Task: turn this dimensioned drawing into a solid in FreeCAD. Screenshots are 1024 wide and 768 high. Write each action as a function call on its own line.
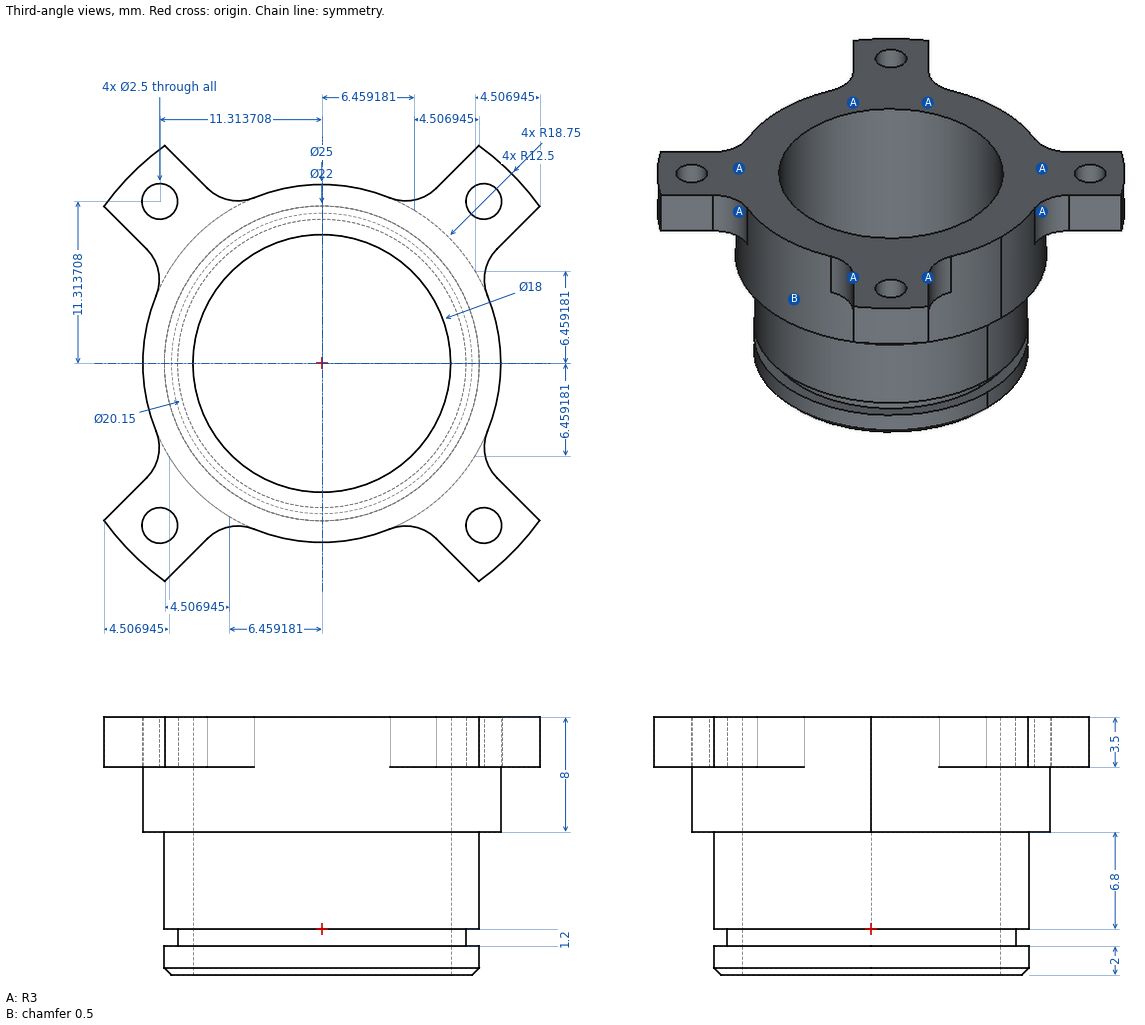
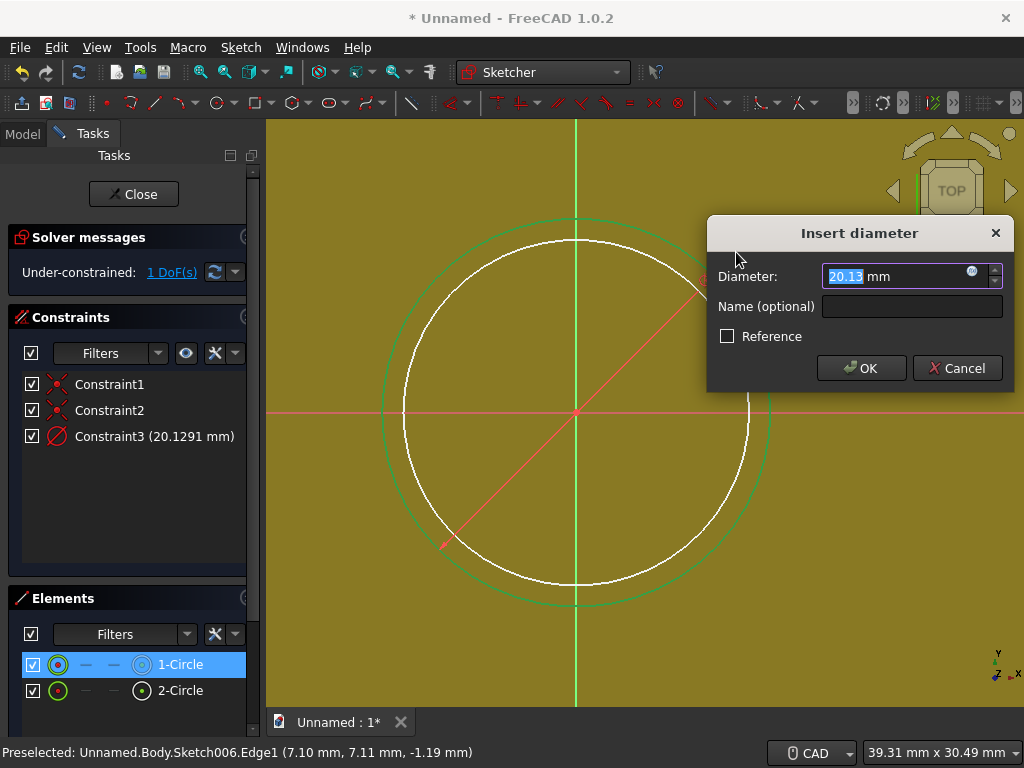
text(20.15)
key(Return)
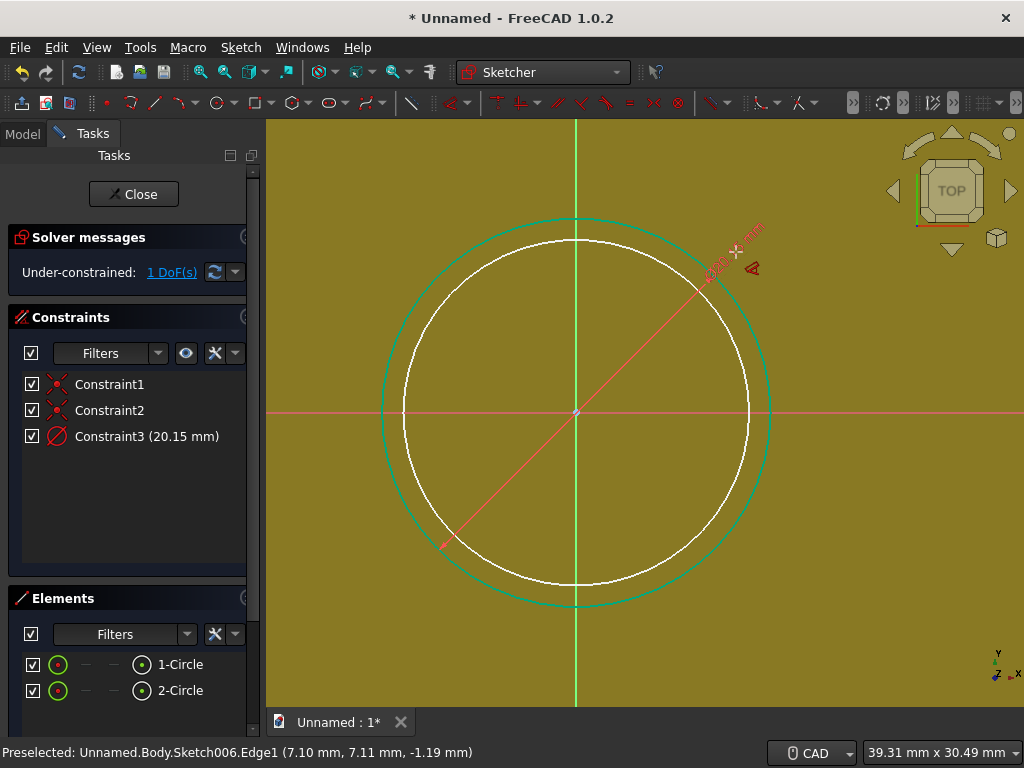
click(698, 290)
click(795, 348)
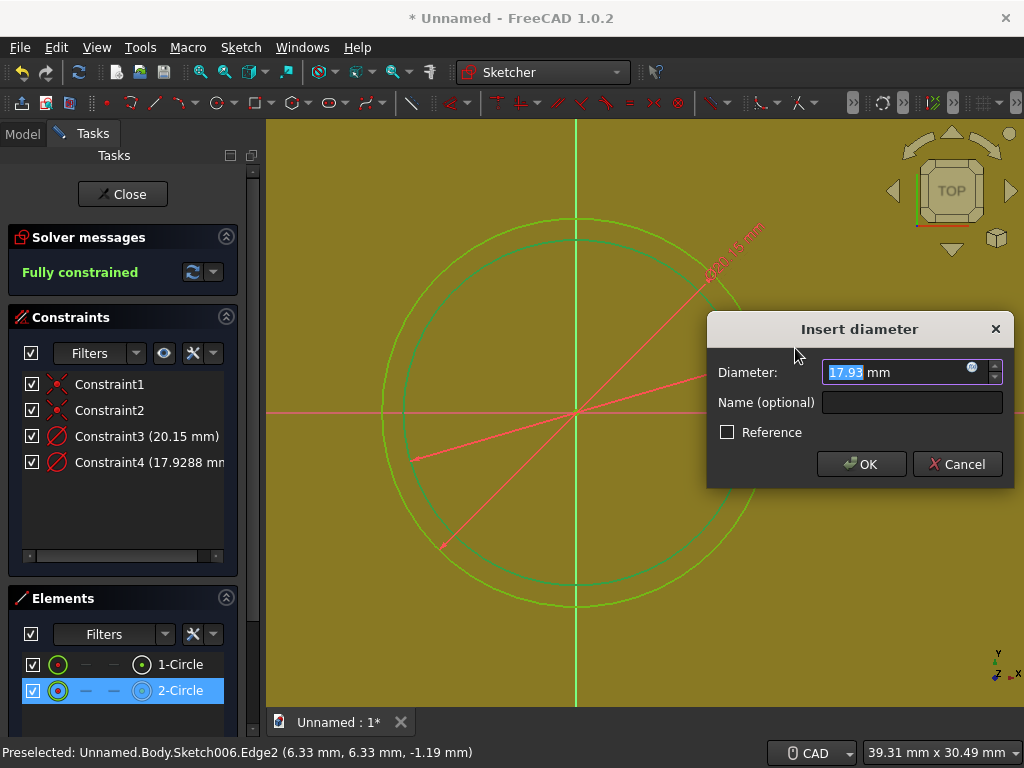
text(18)
key(Return)
key(Escape)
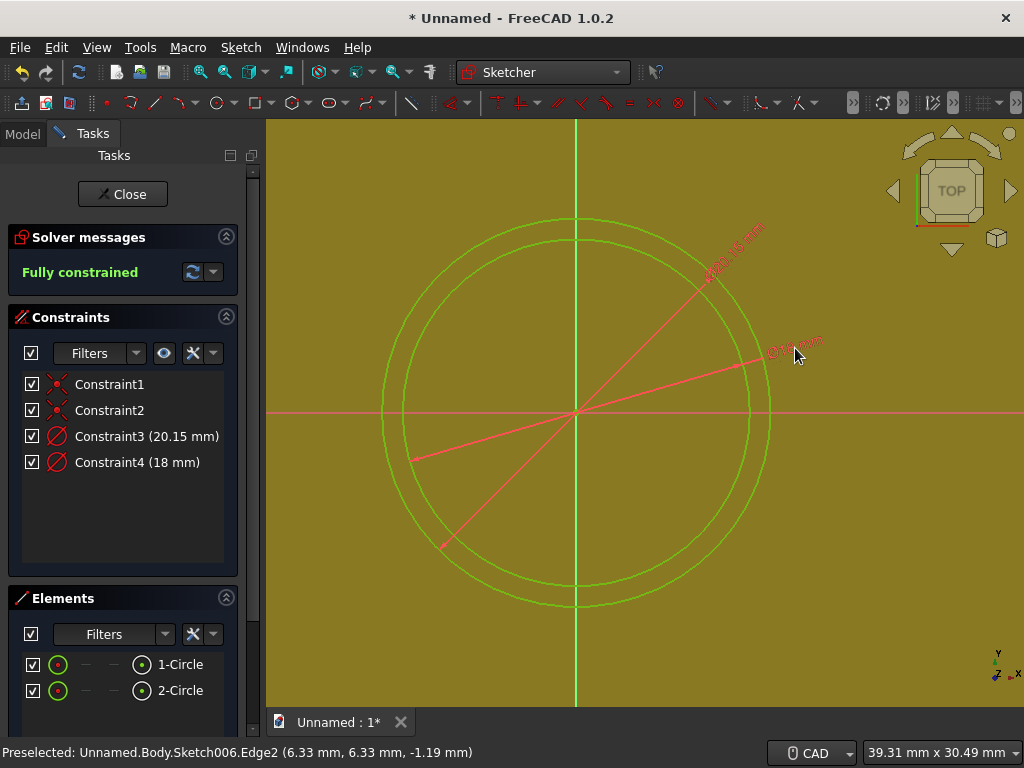
click(123, 194)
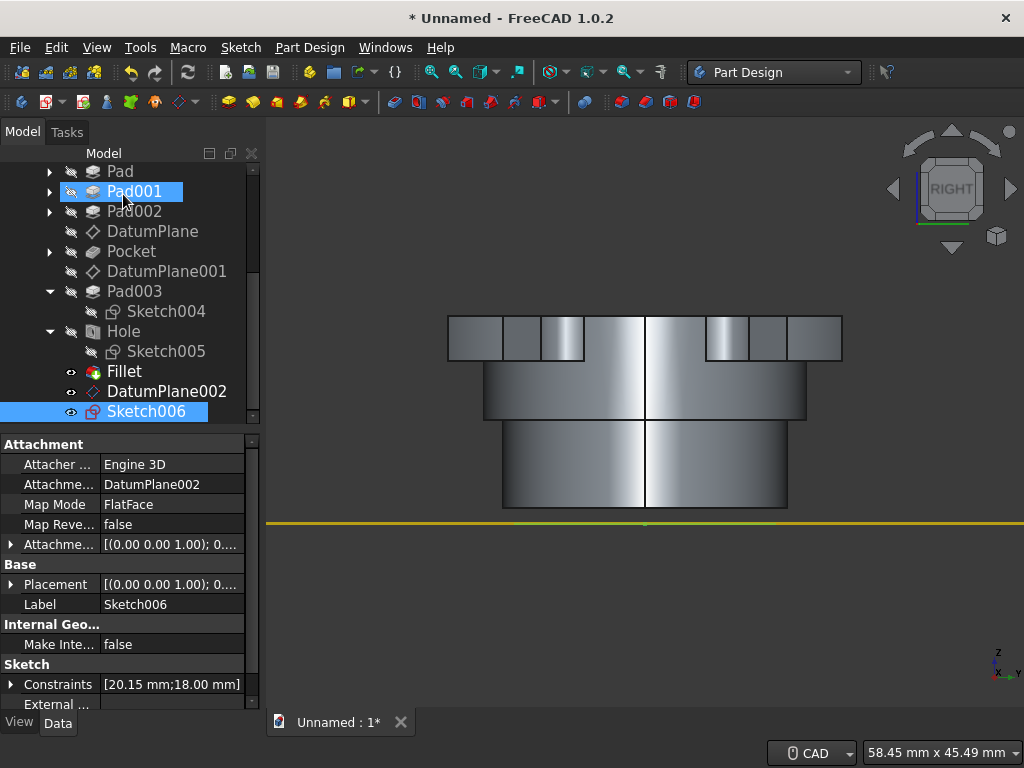
click(230, 102)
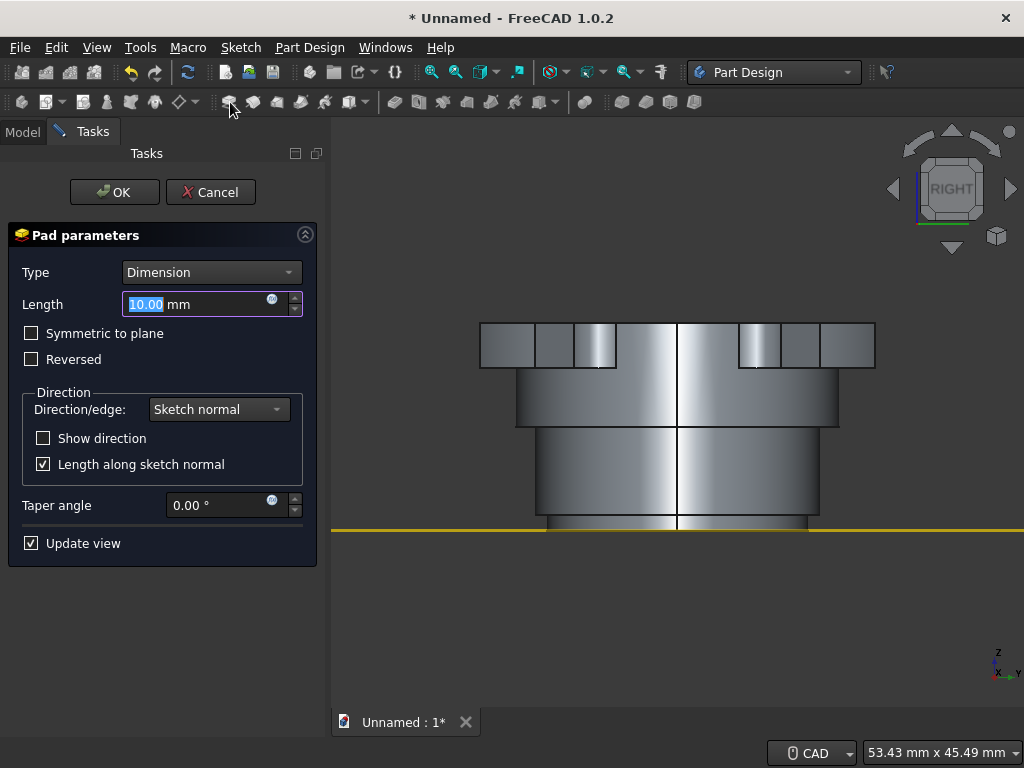
text(1.2)
key(Tab)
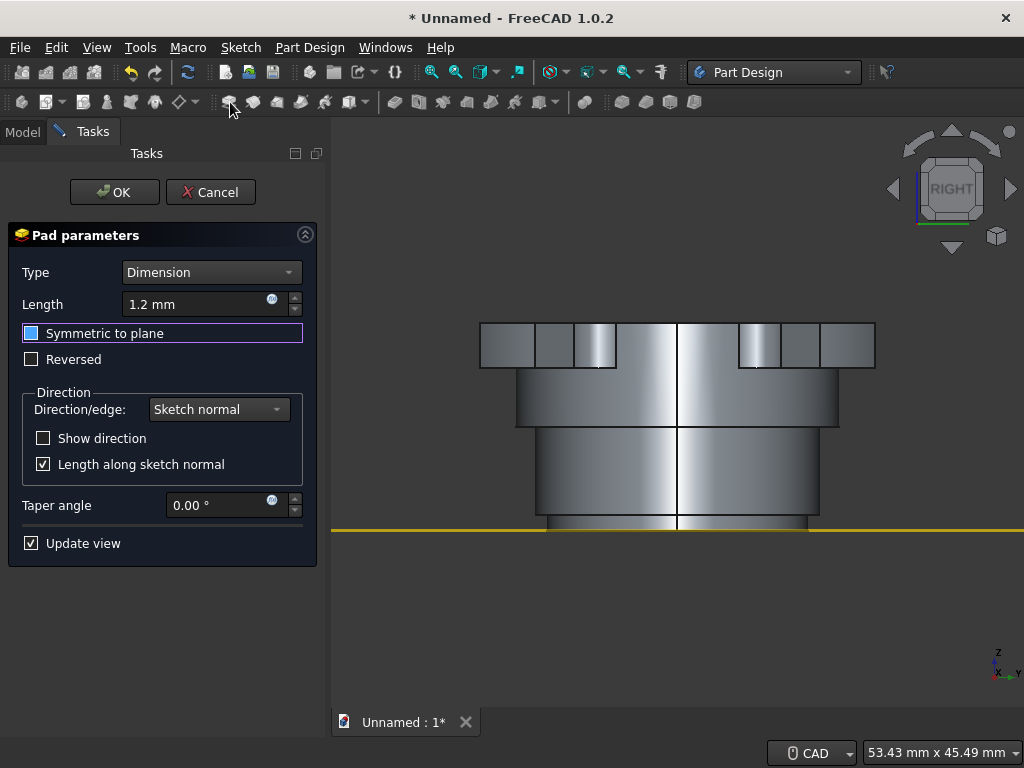
click(115, 192)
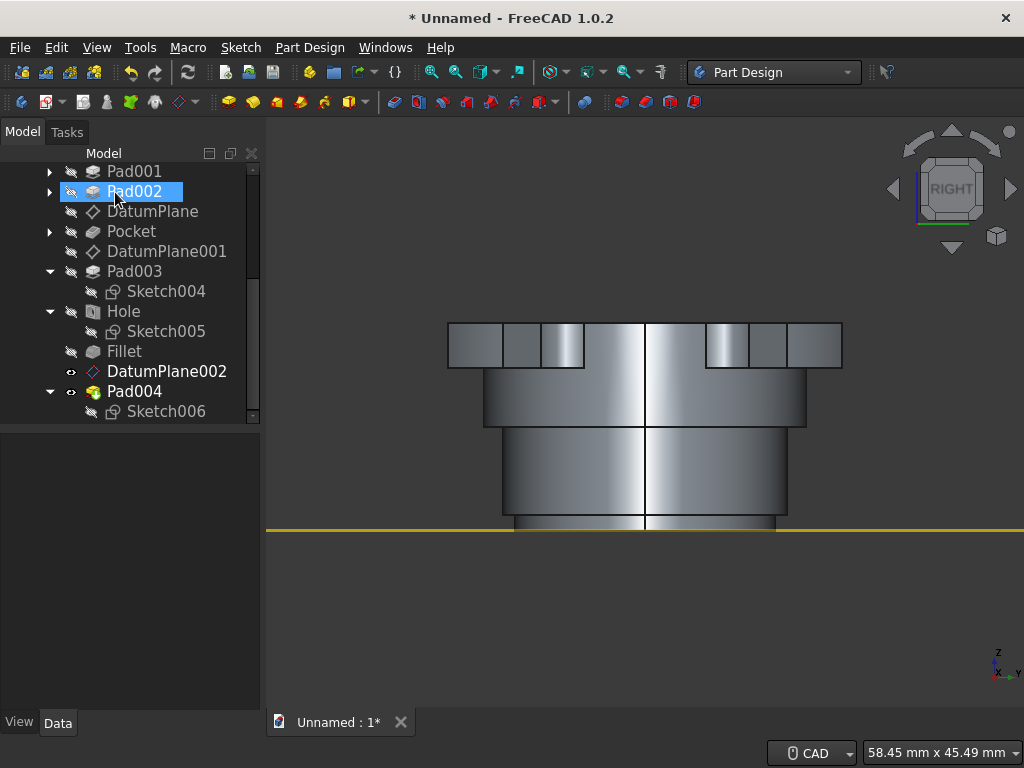
click(116, 372)
key(space)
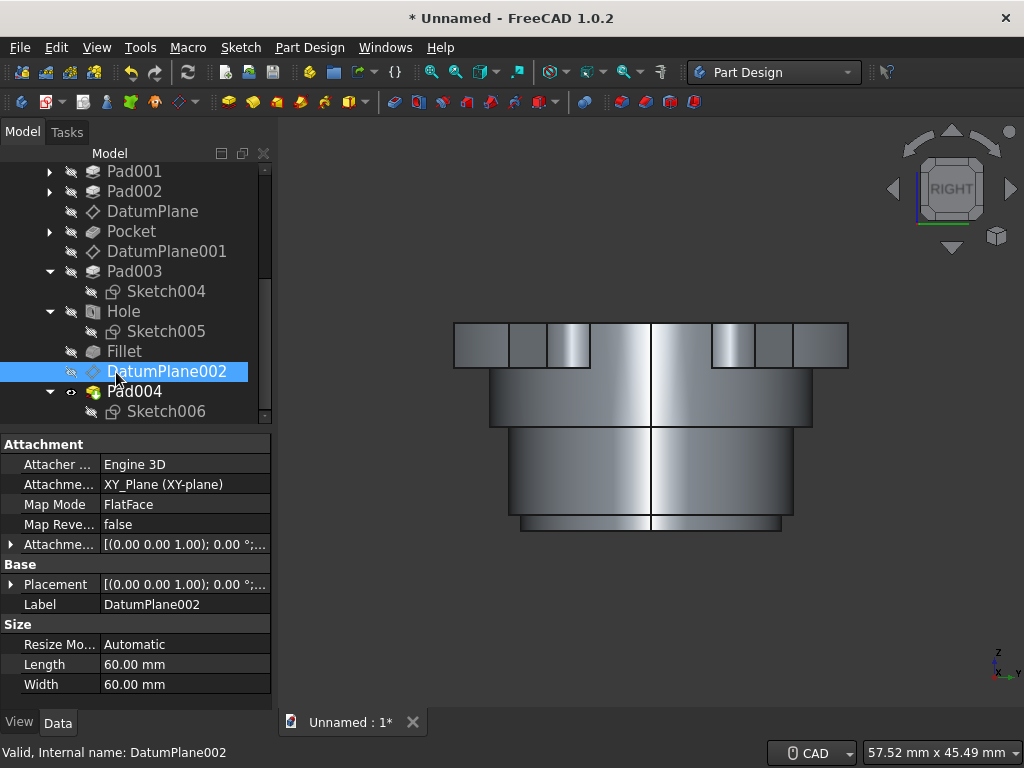
scroll(140, 287, down, 3)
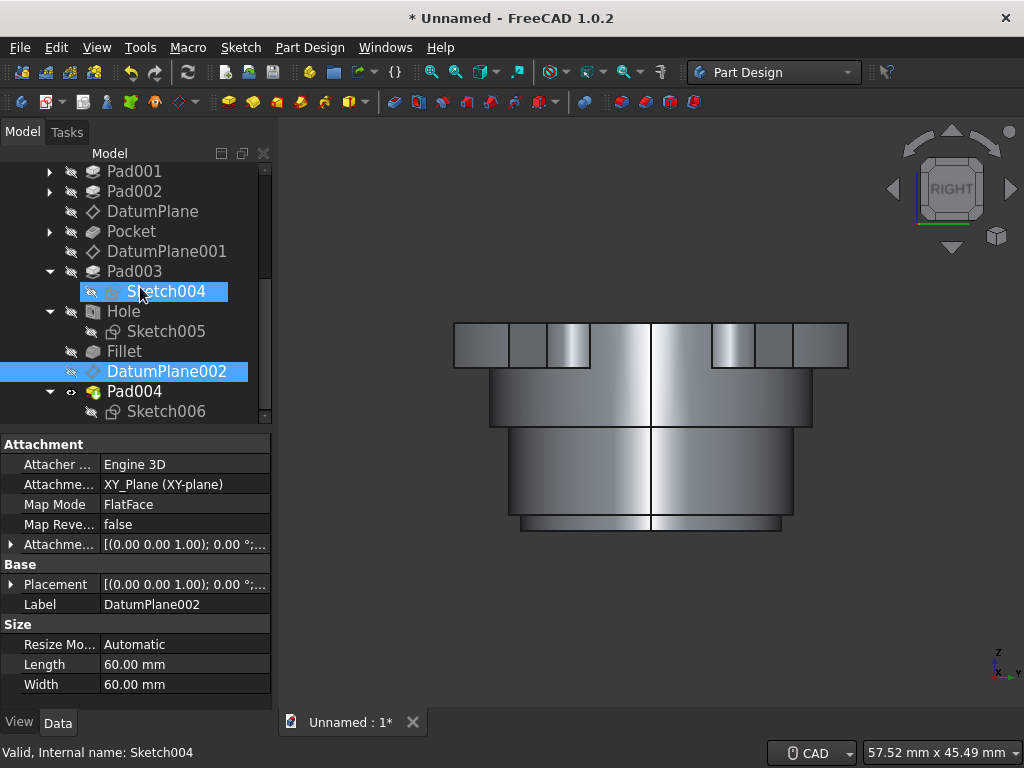
scroll(140, 287, up, 15)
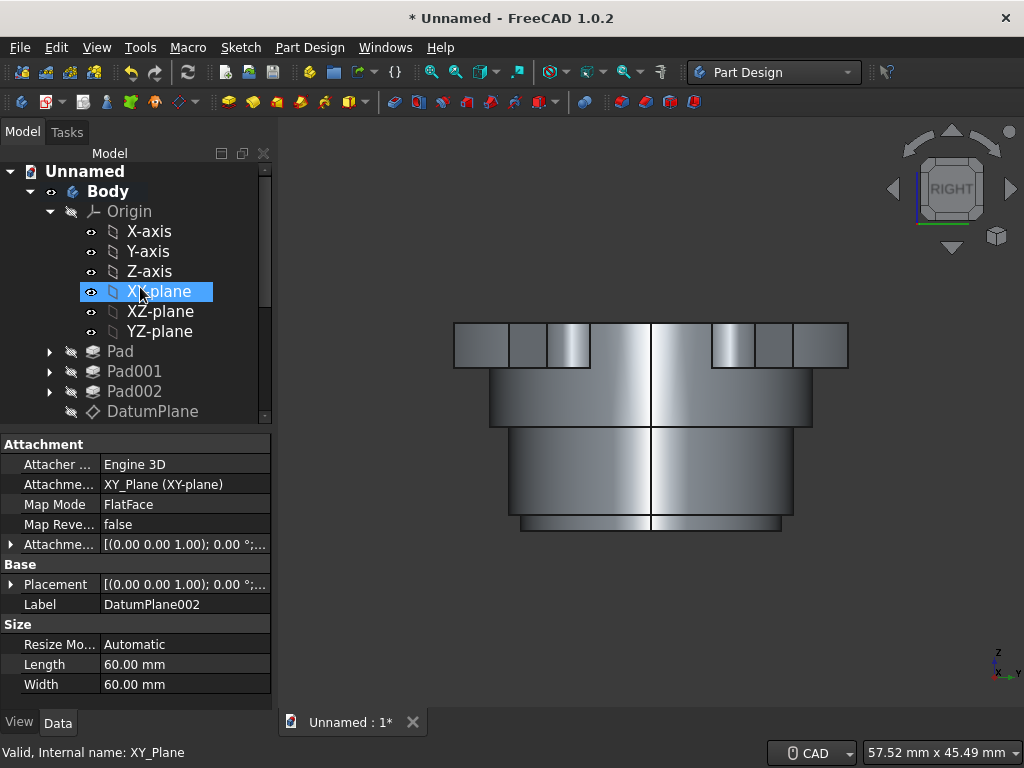
click(136, 292)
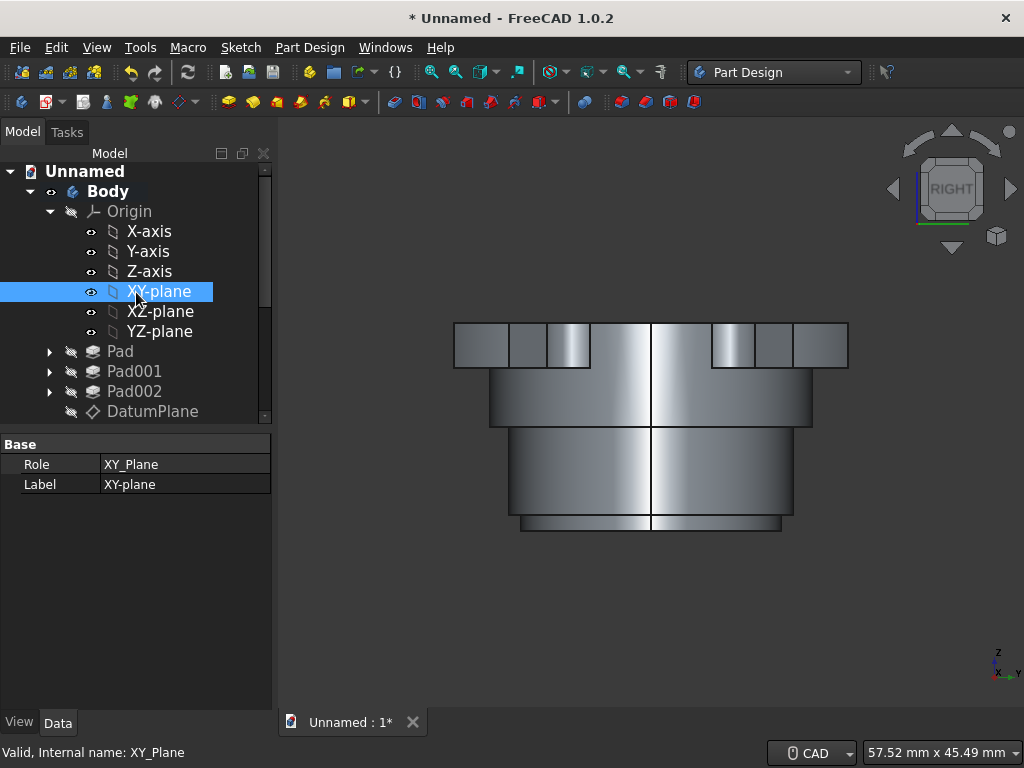
click(180, 102)